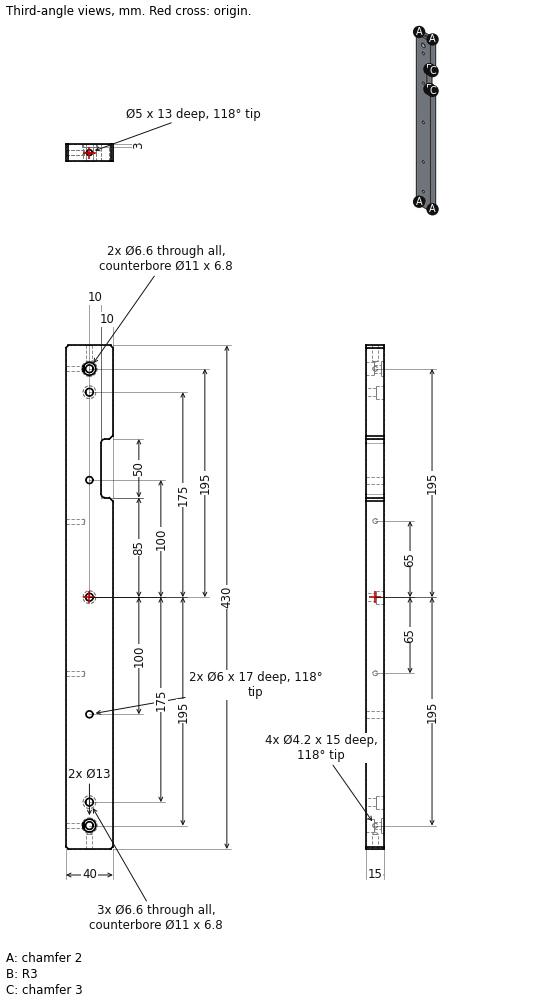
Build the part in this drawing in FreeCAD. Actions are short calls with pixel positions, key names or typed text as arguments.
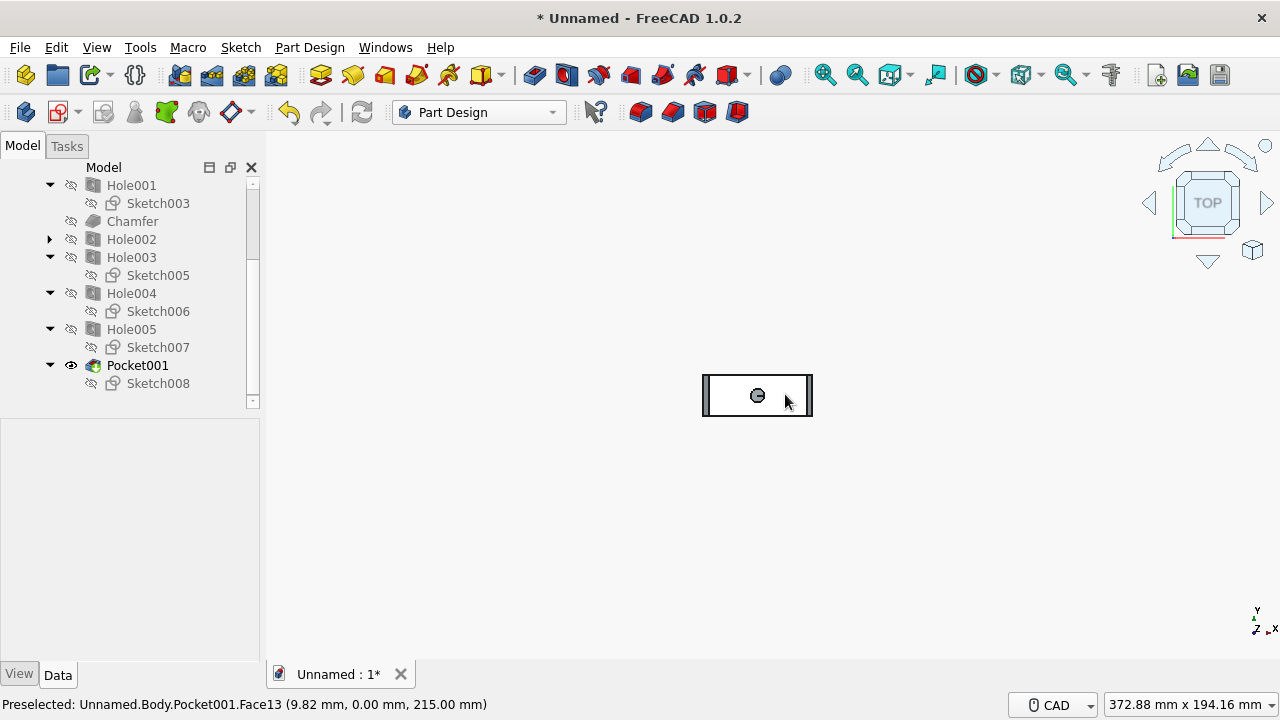
click(826, 76)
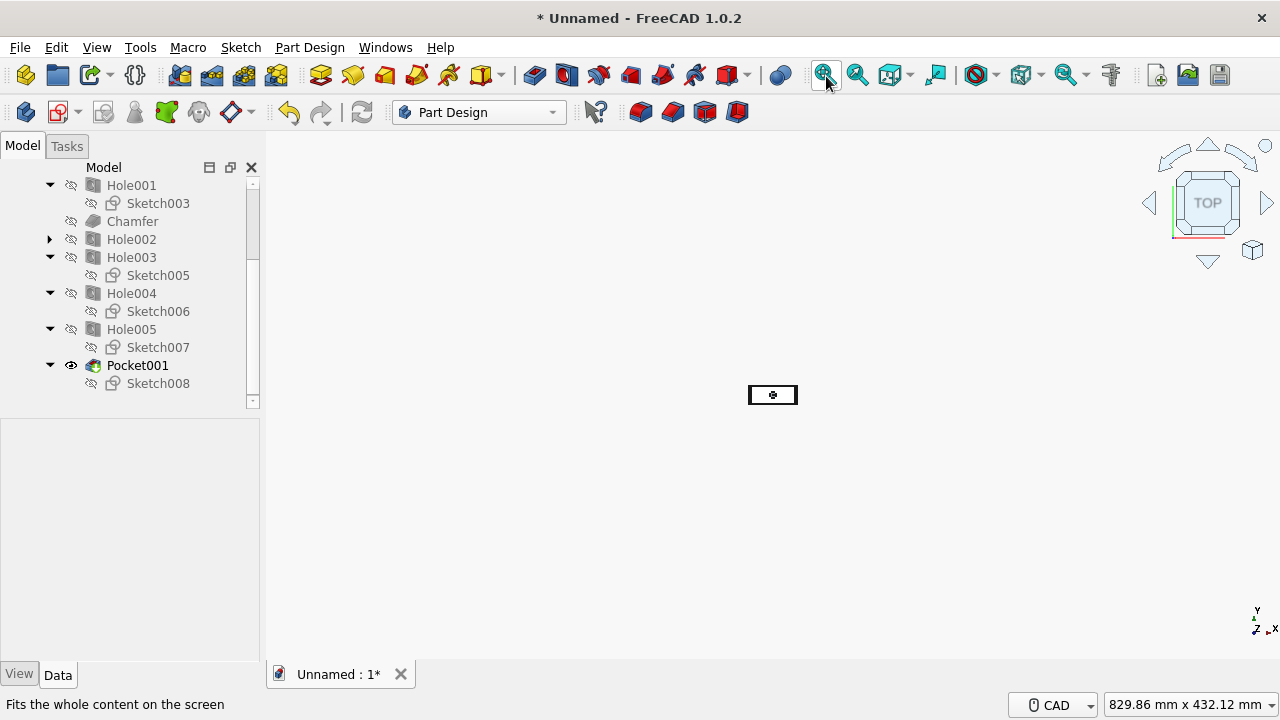
key(0)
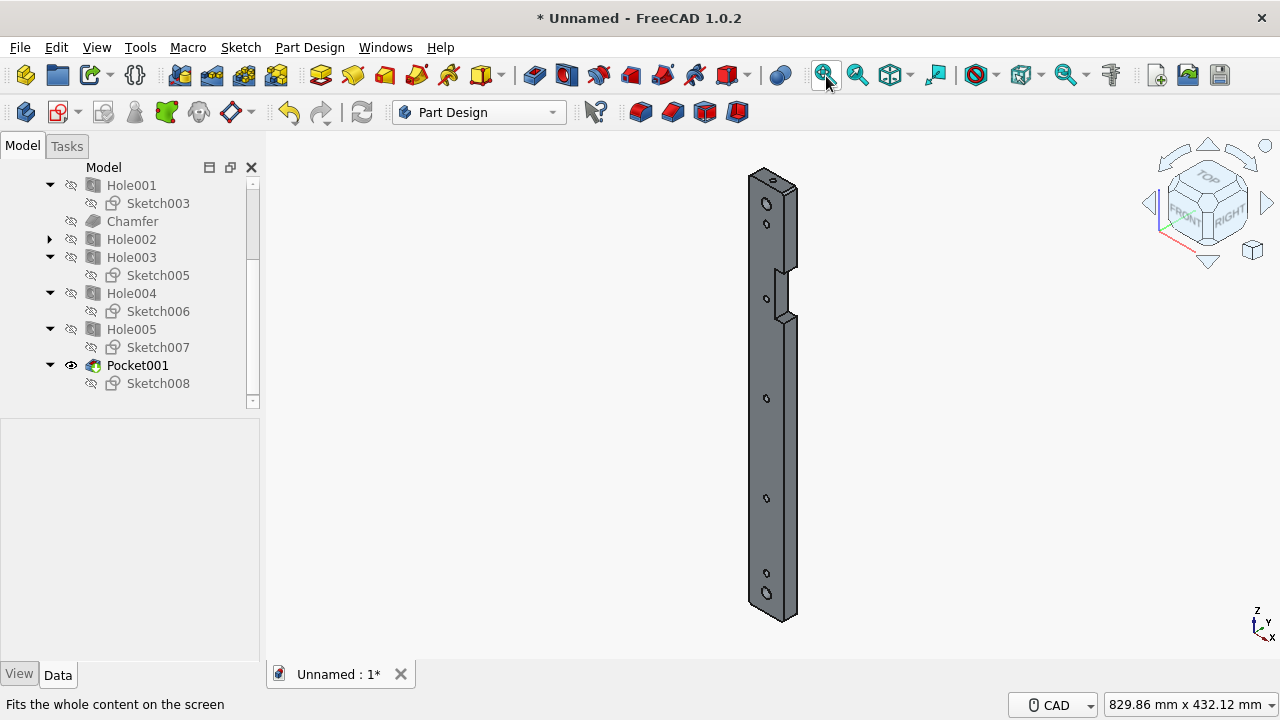
scroll(782, 314, up, 4)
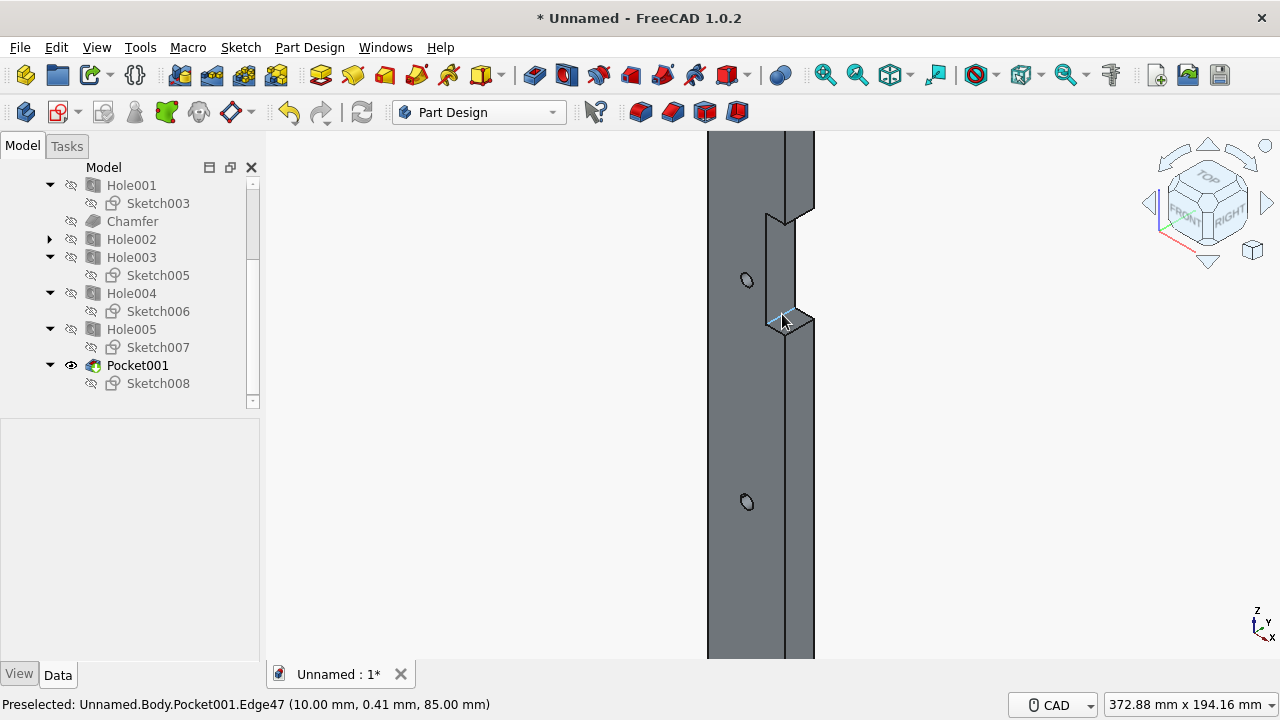
click(826, 76)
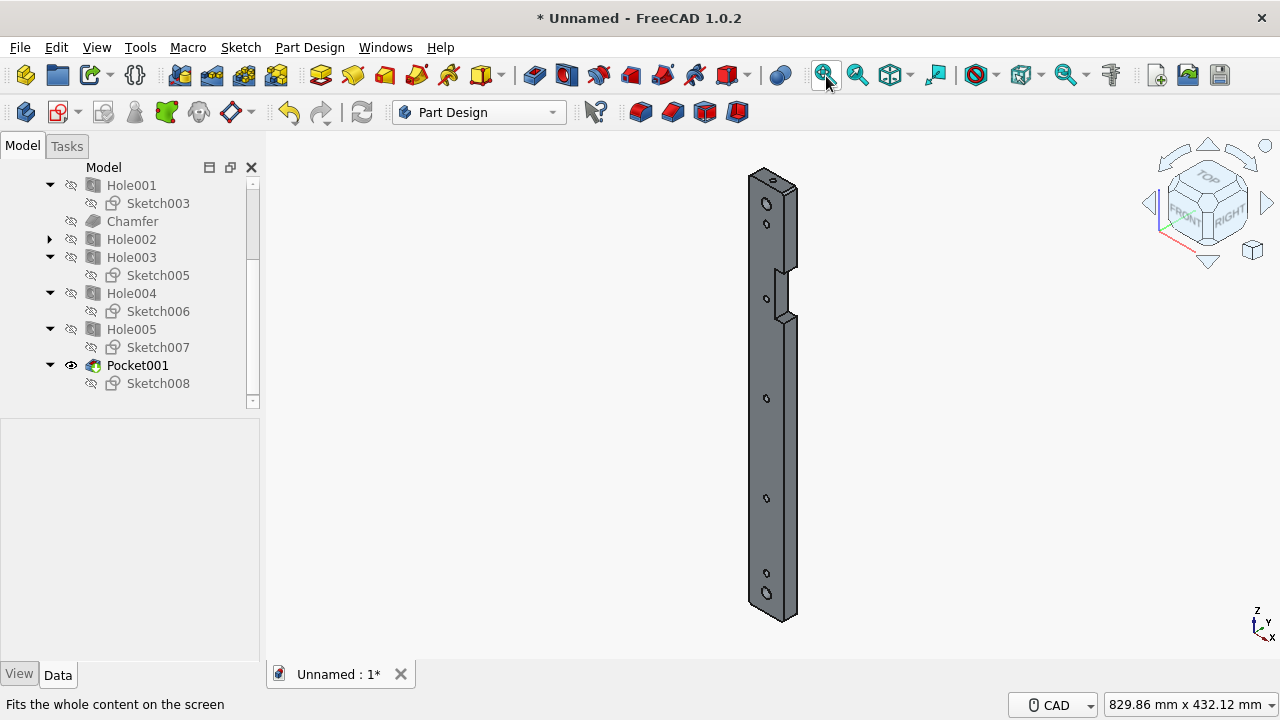
key(1)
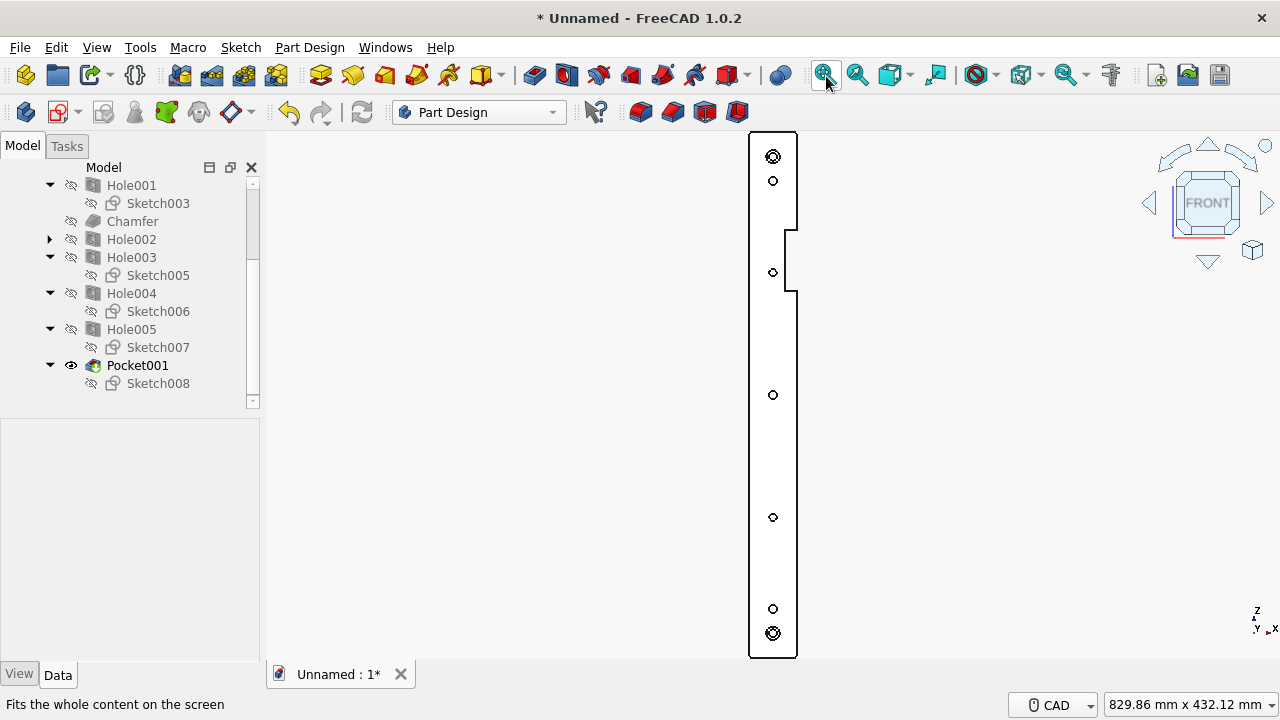
scroll(785, 290, up, 4)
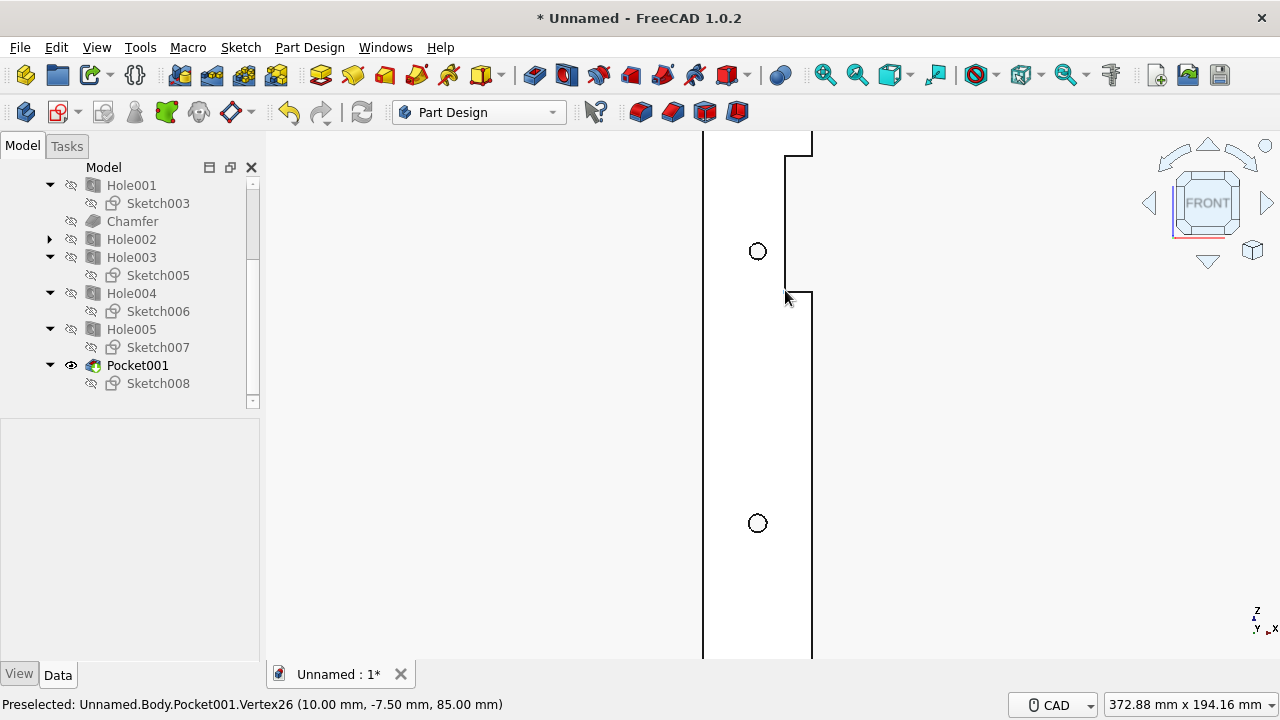
click(826, 76)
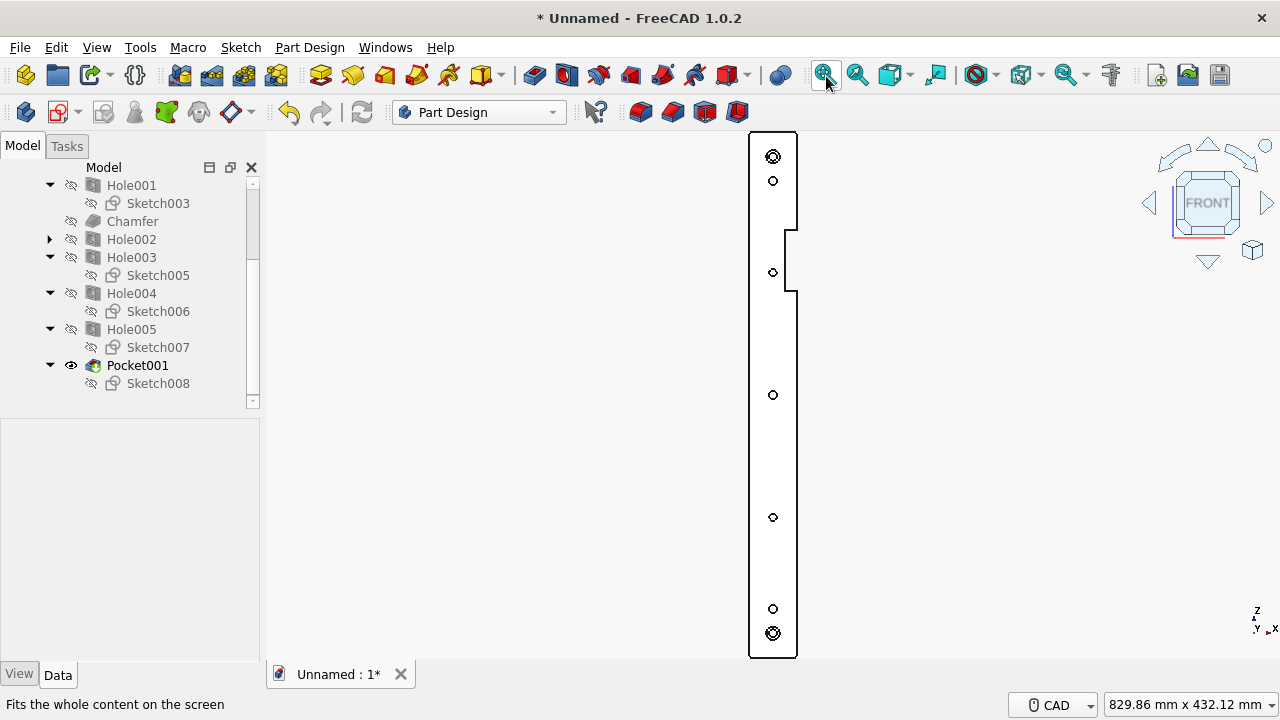
key(3)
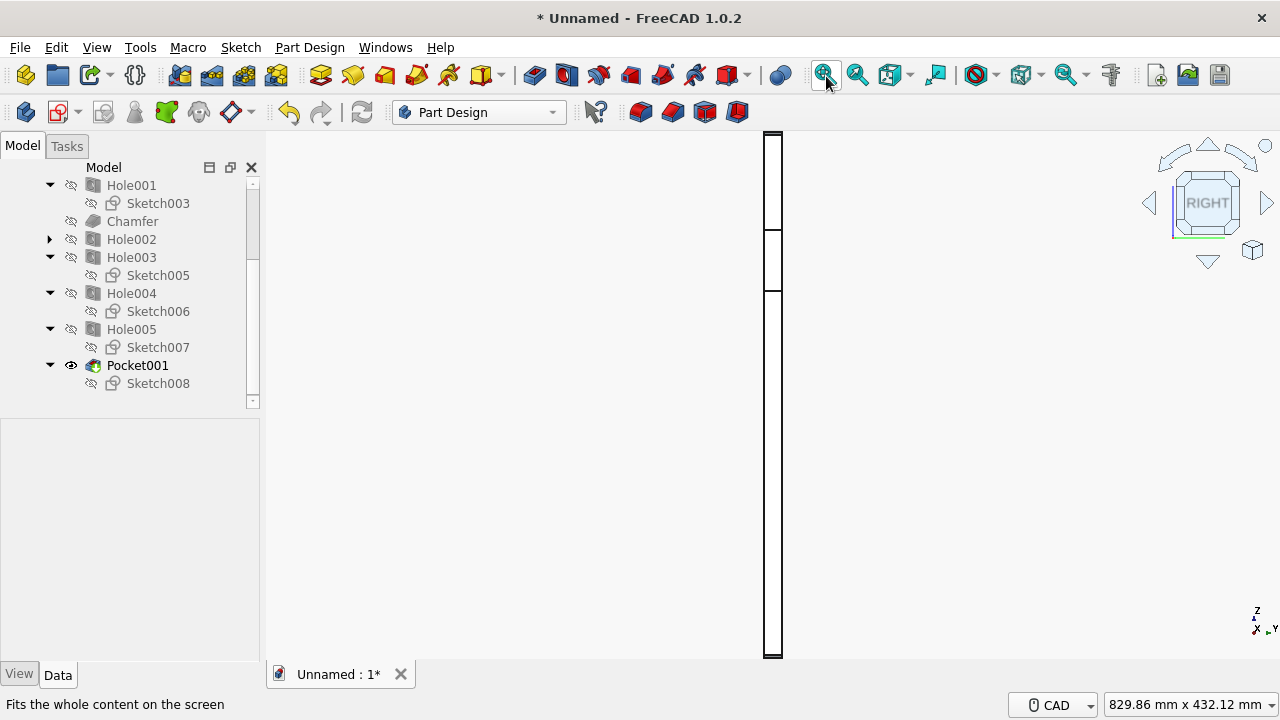
scroll(773, 290, up, 4)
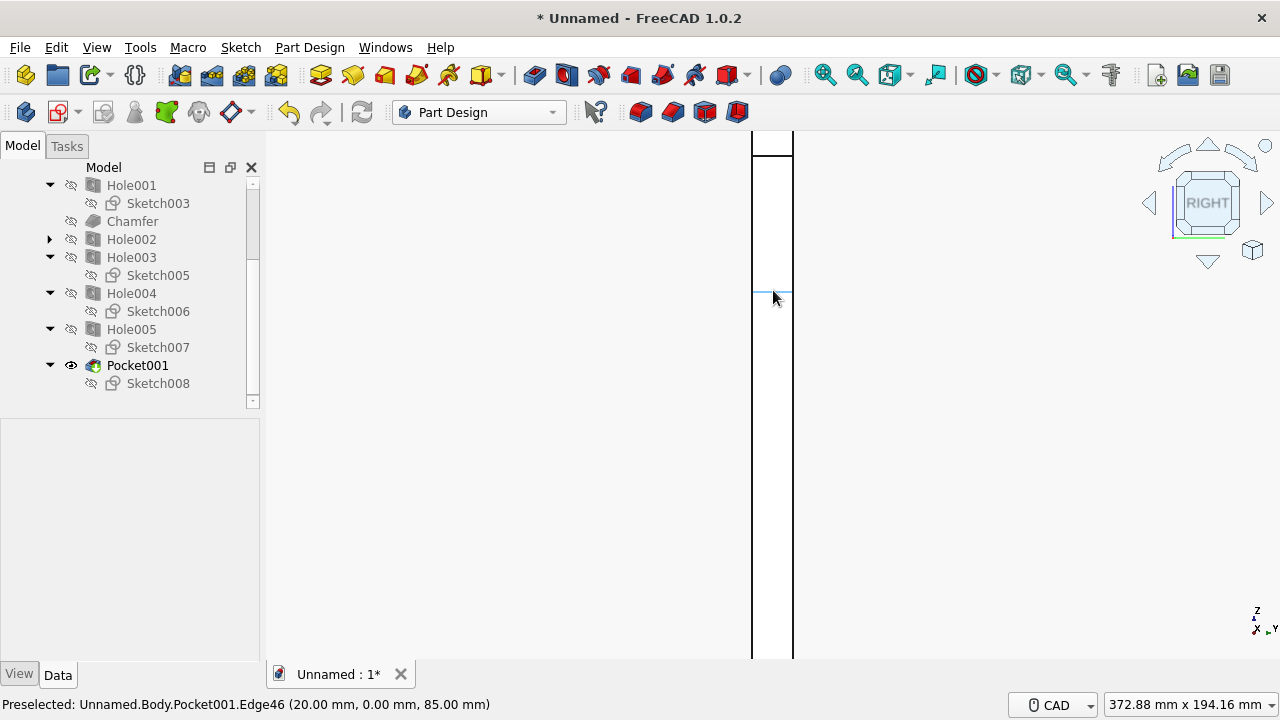
click(826, 76)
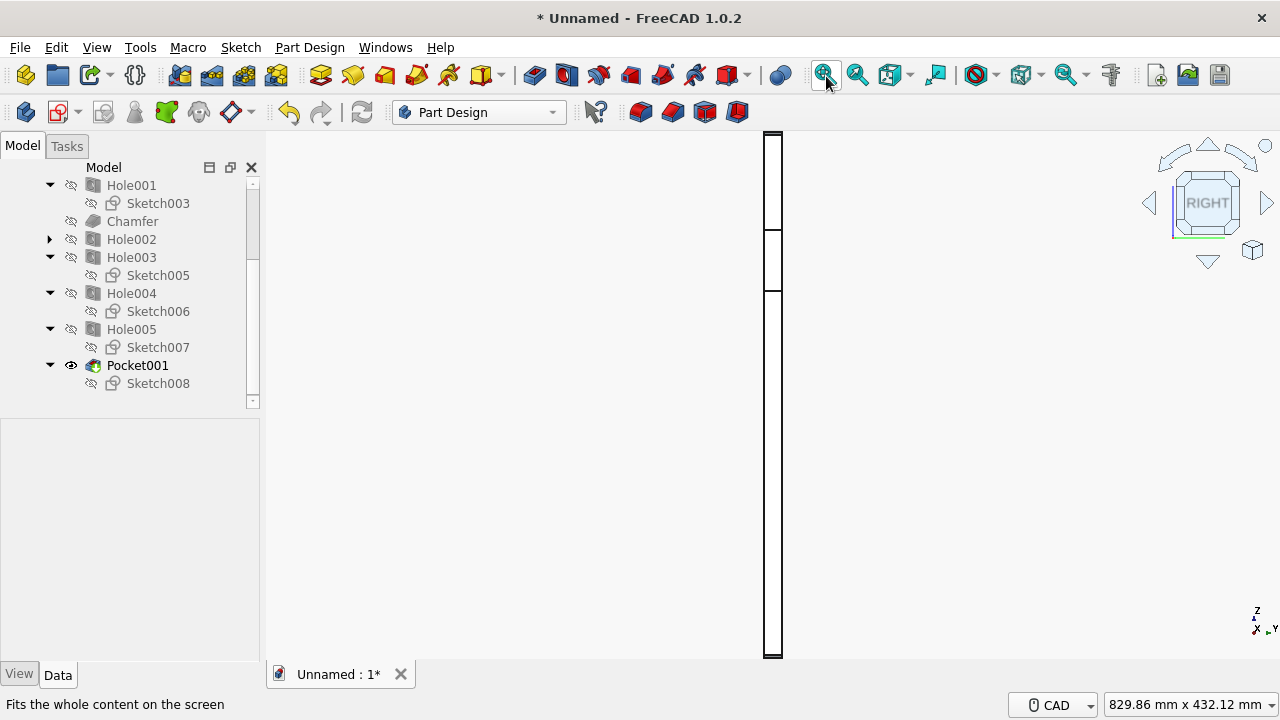
key(5)